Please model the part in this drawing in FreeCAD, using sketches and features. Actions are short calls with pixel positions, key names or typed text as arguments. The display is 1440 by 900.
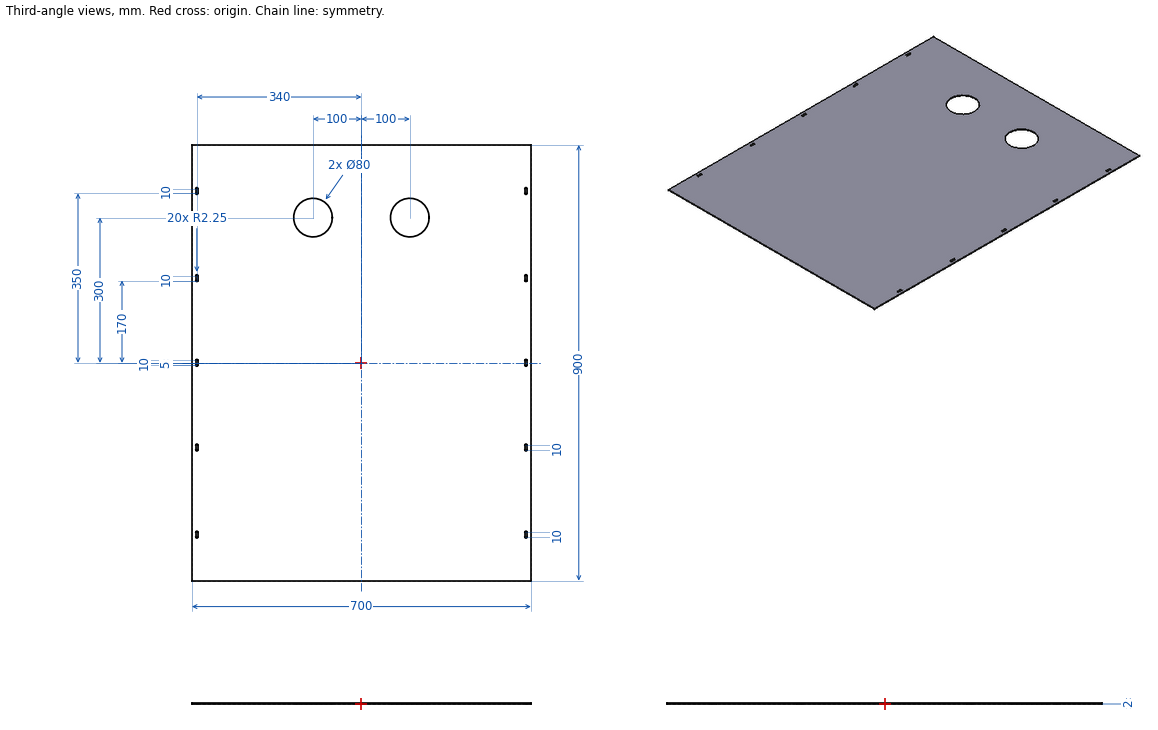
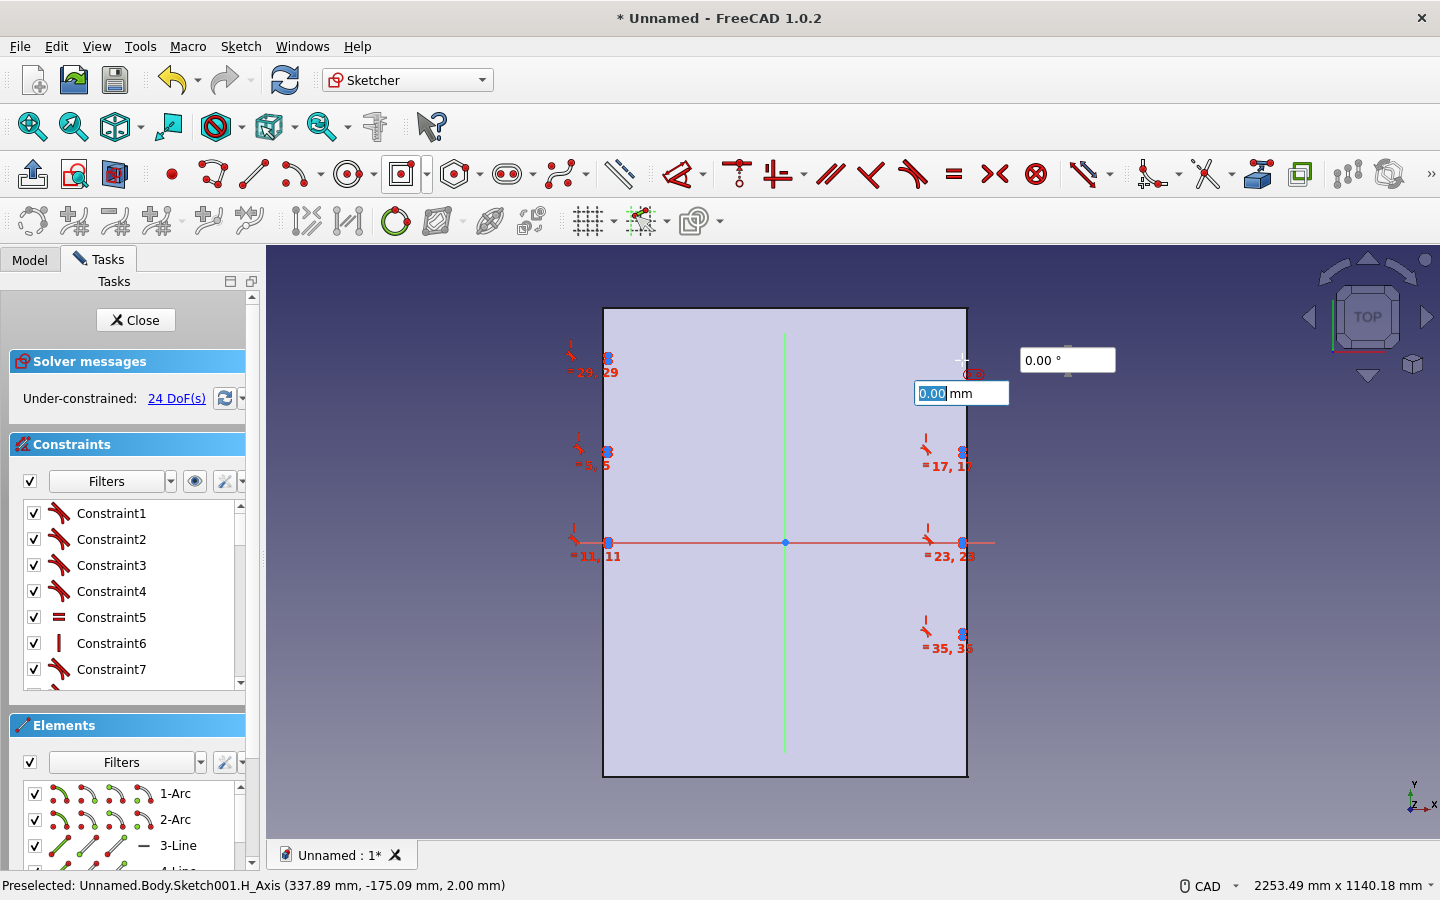
scroll(962, 355, up, 6)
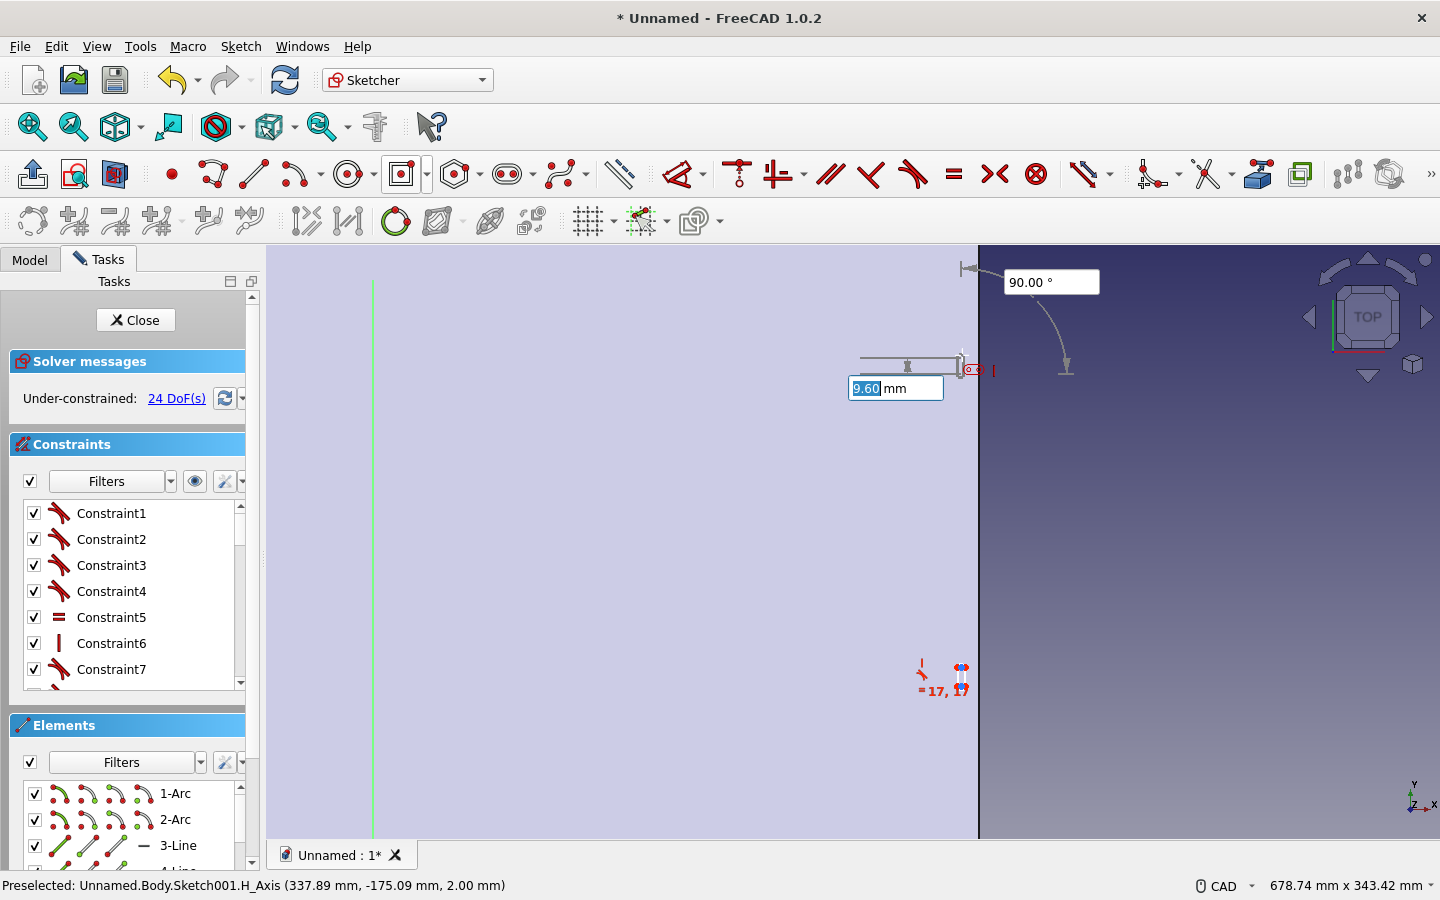
click(961, 355)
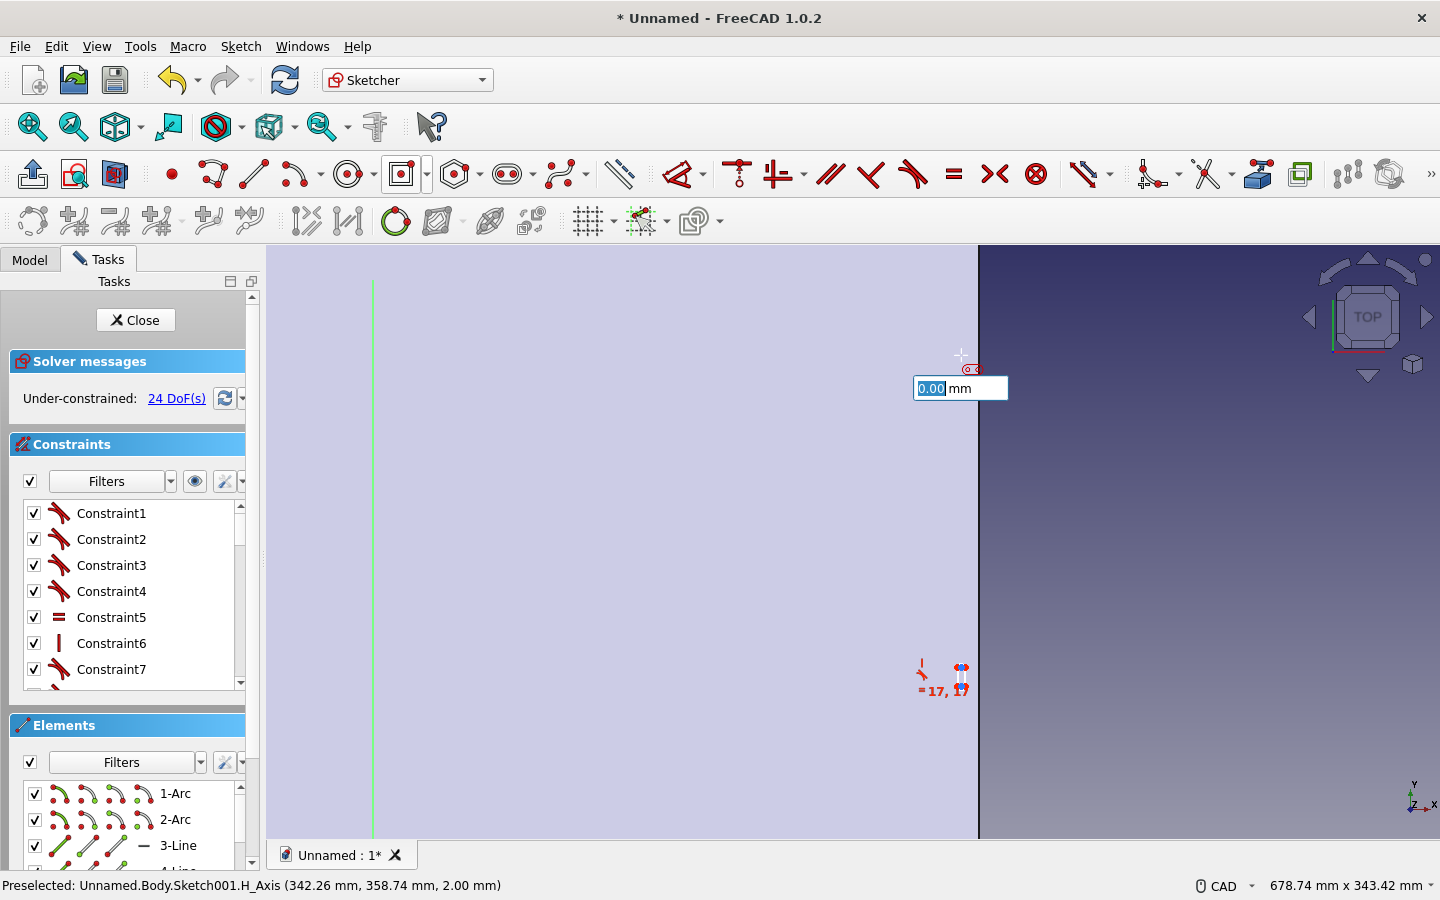
scroll(965, 364, up, 8)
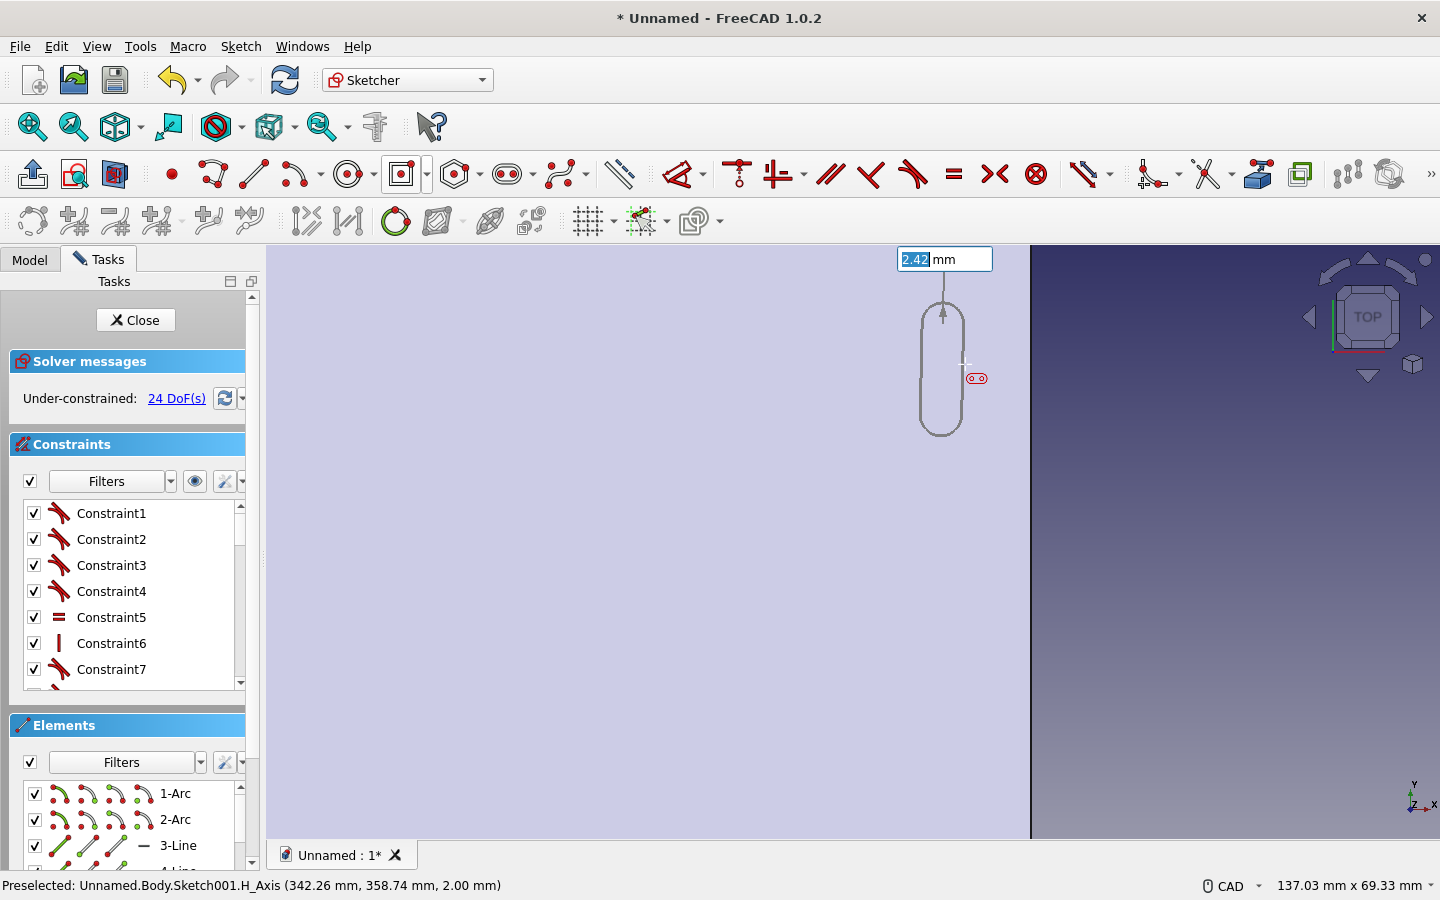
click(965, 361)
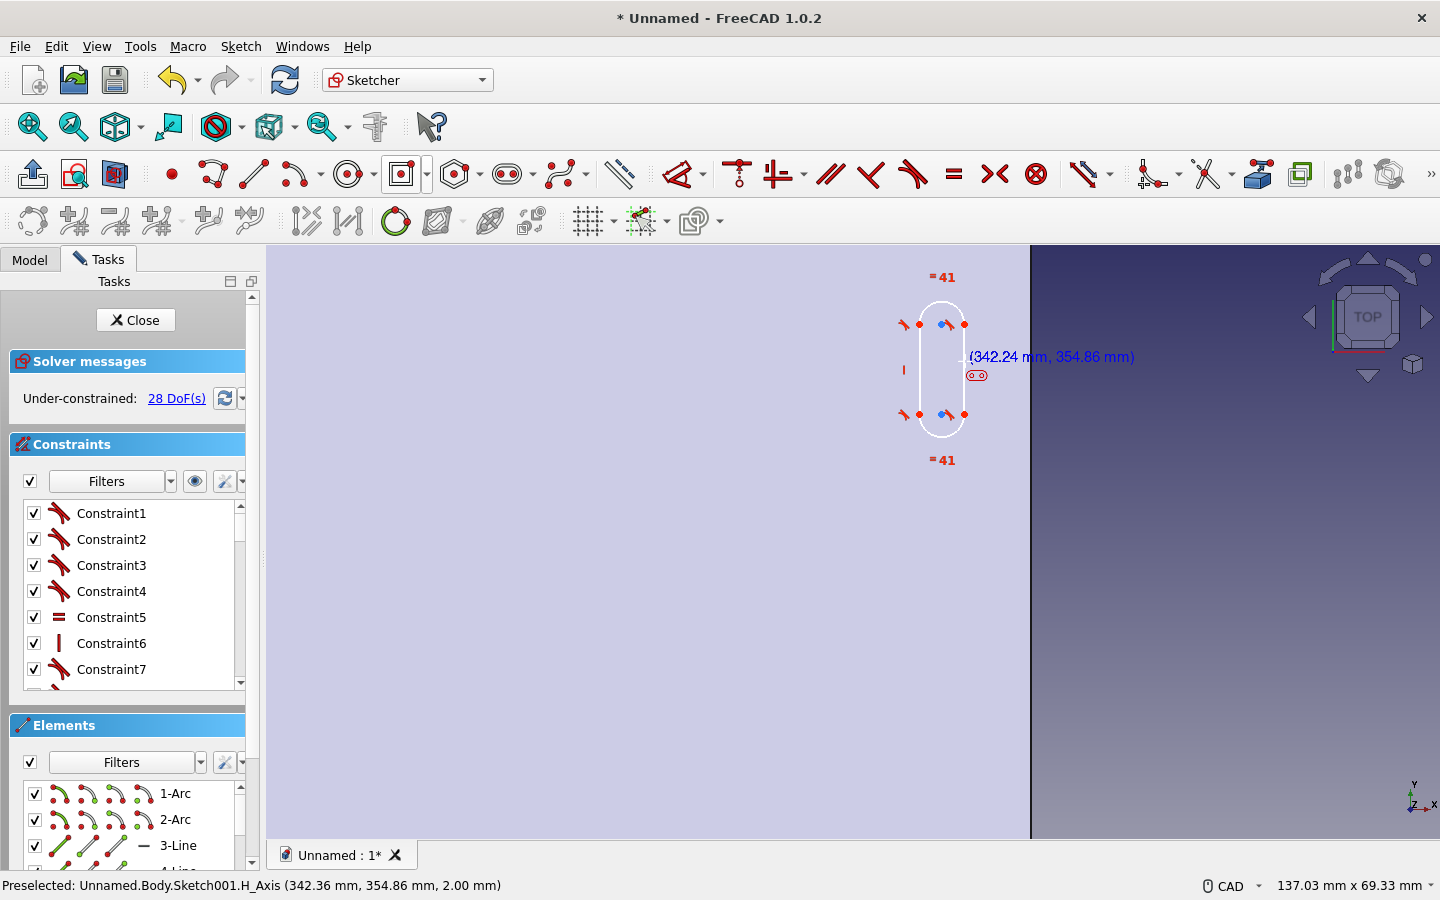
scroll(963, 357, down, 14)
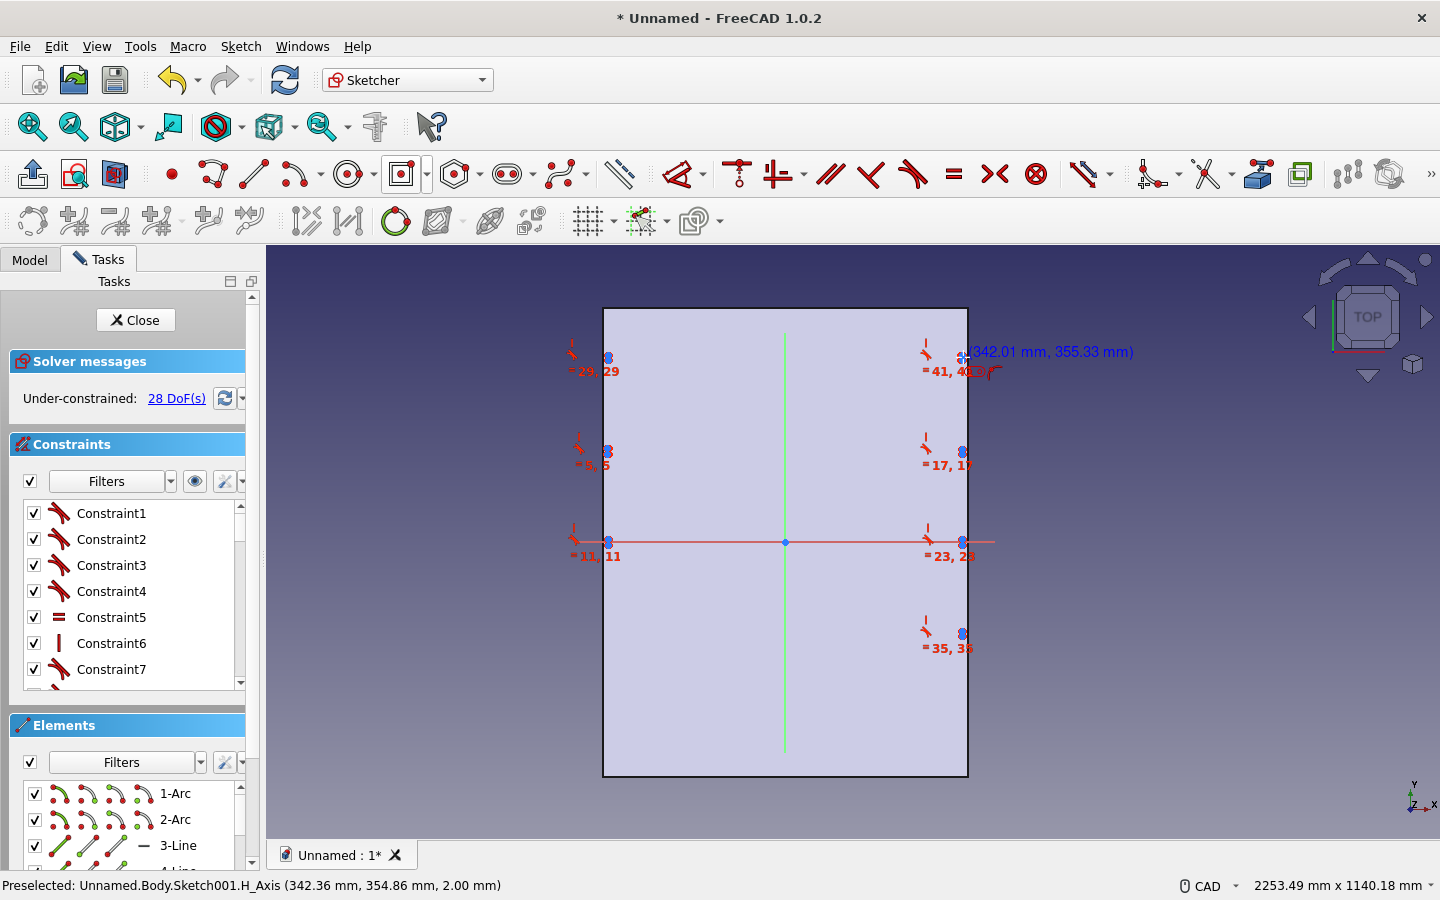
scroll(963, 730, up, 15)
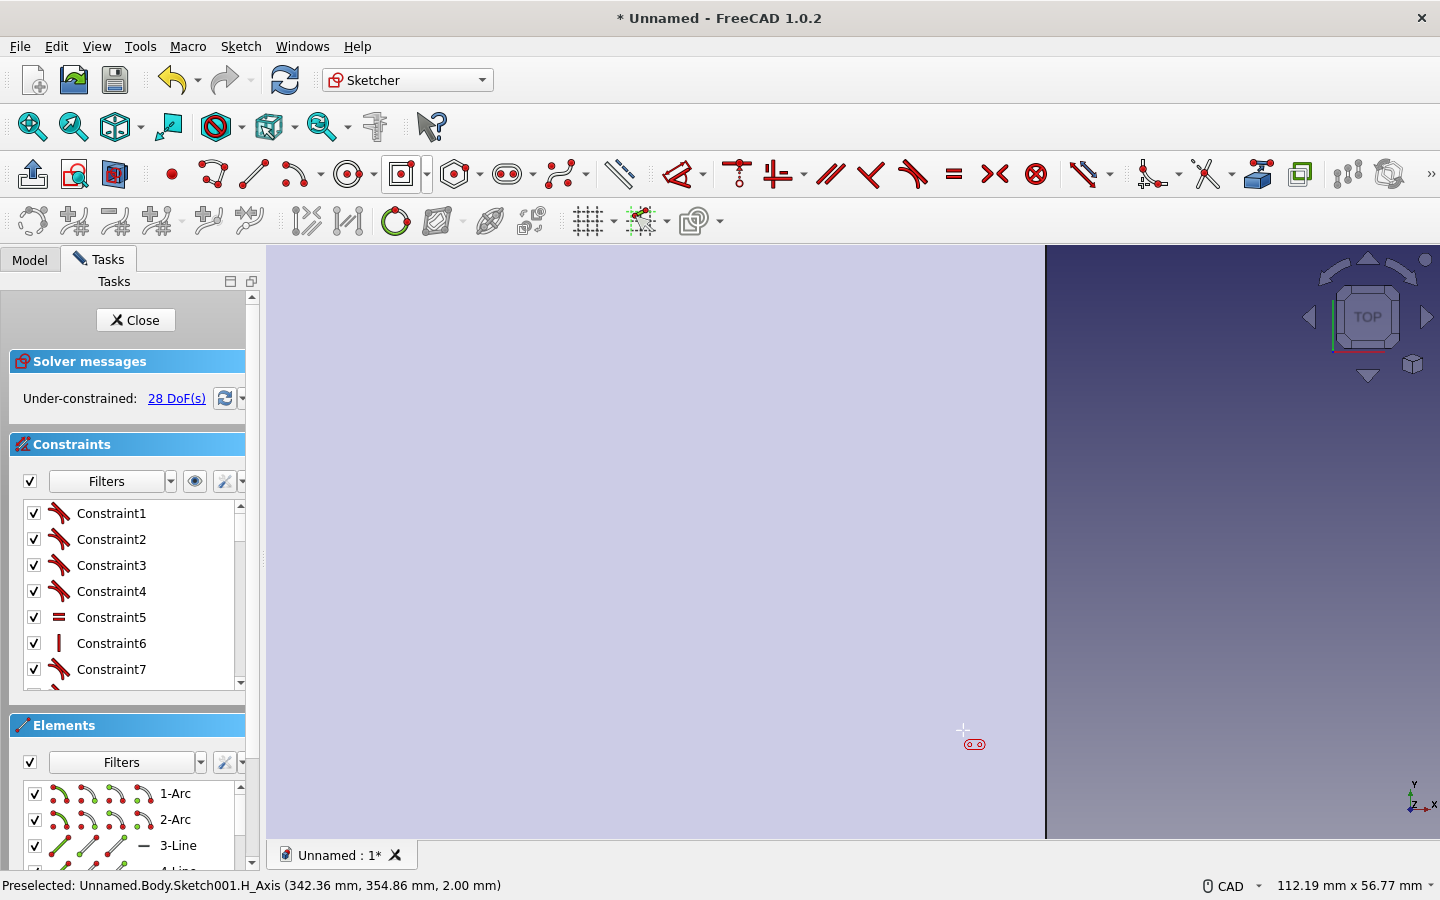
scroll(963, 730, down, 15)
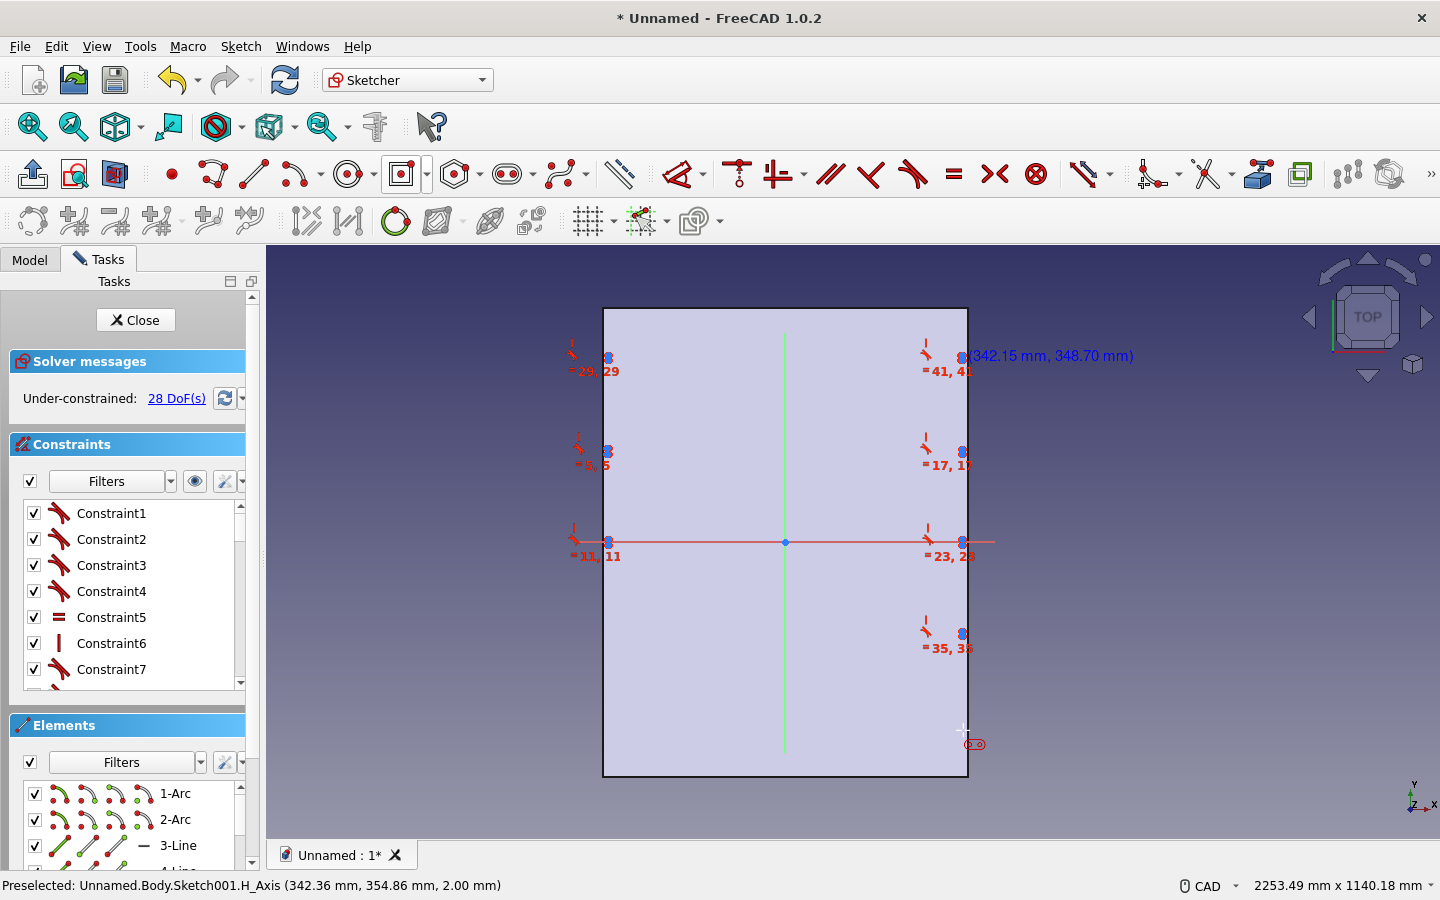
click(963, 730)